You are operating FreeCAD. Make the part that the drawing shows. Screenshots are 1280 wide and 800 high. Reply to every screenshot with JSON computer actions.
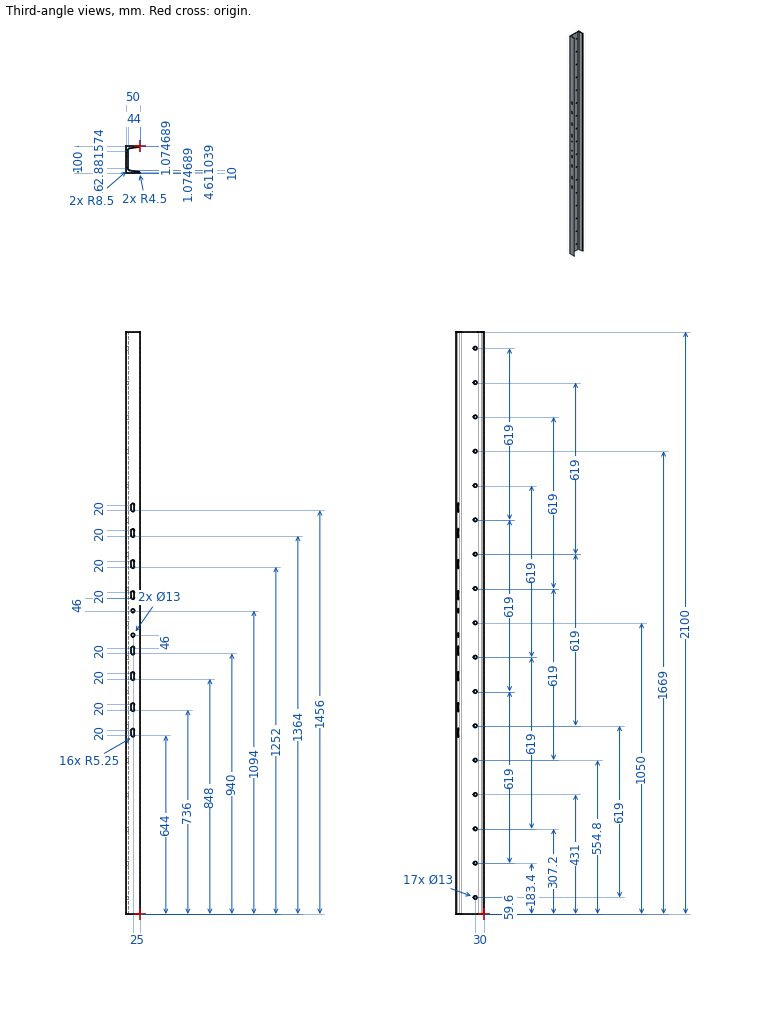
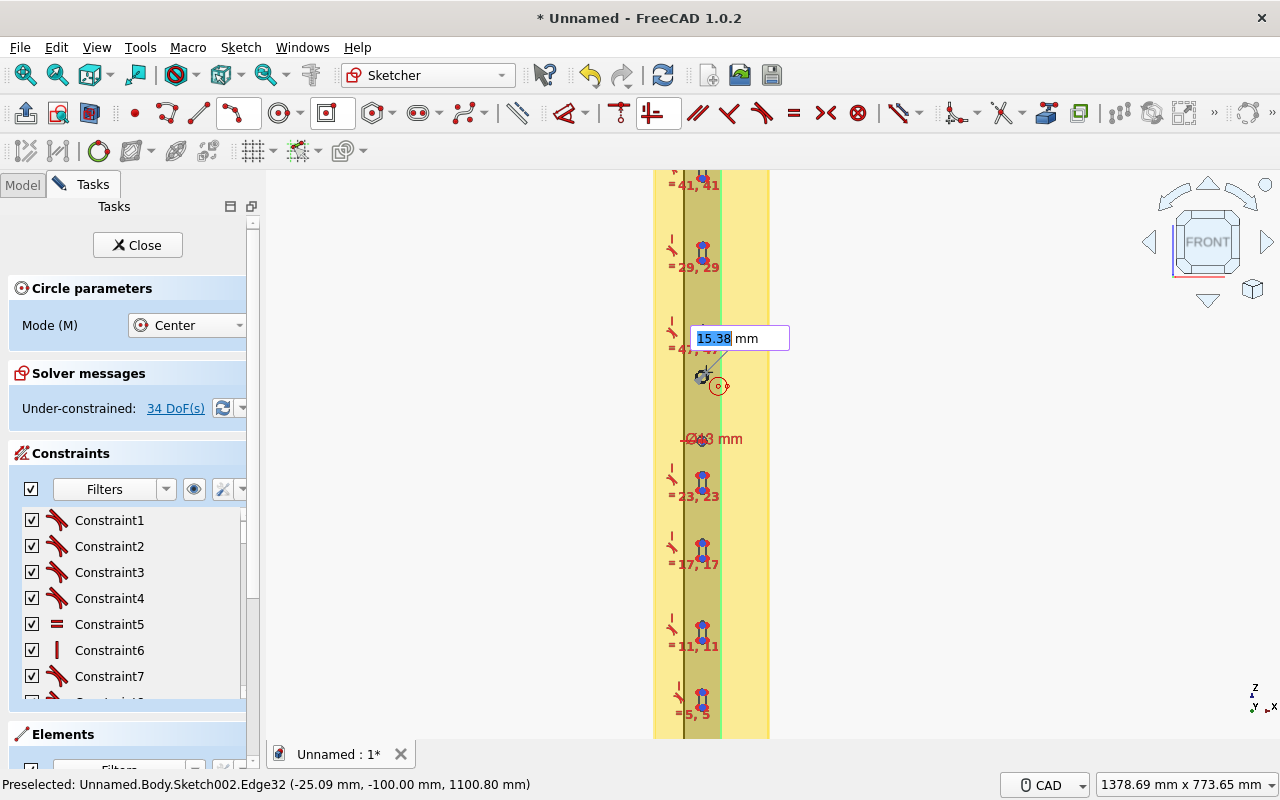
{"action": "type", "text": "13"}
{"action": "key", "text": "Return"}
{"action": "key", "text": "Escape"}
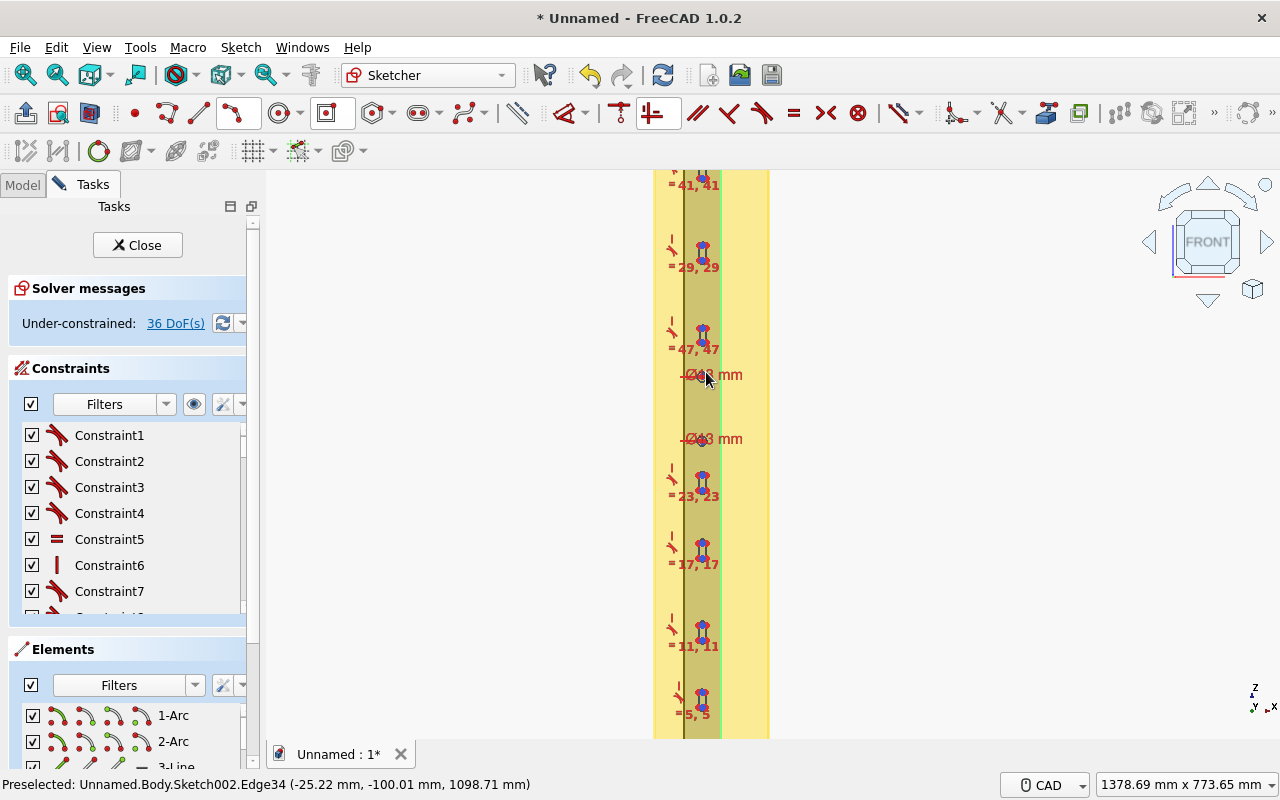
{"action": "scroll", "coordinate": [702, 376], "scroll_direction": "down", "scroll_amount": 6}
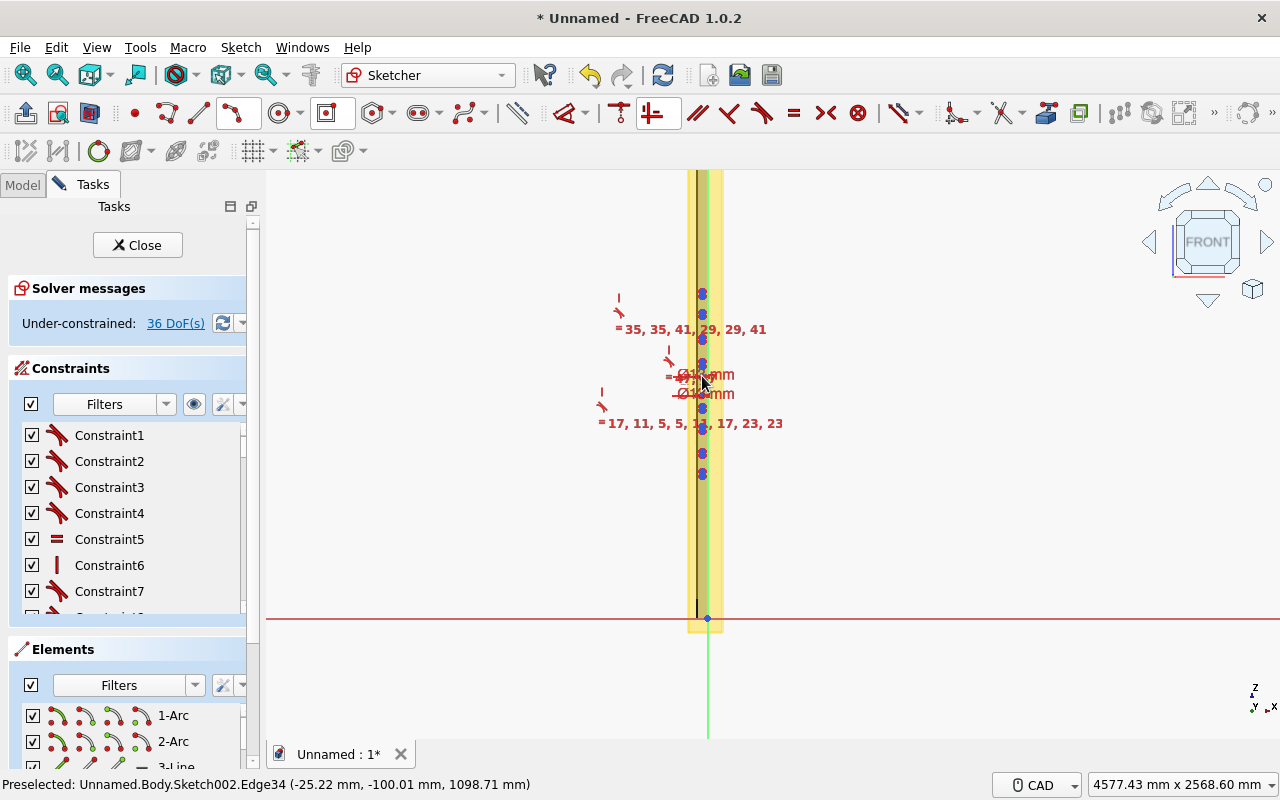
{"action": "scroll", "coordinate": [702, 477], "scroll_direction": "up", "scroll_amount": 13}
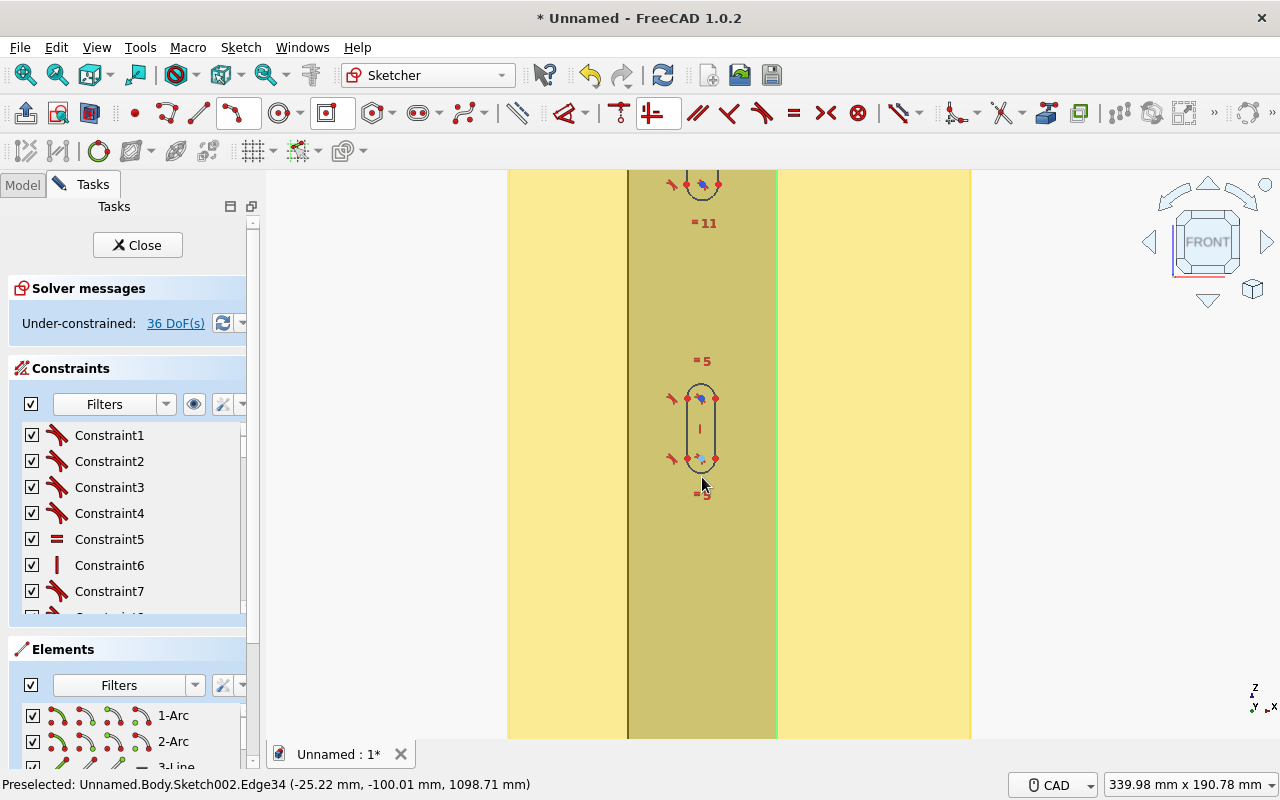
{"action": "left_click", "coordinate": [701, 473]}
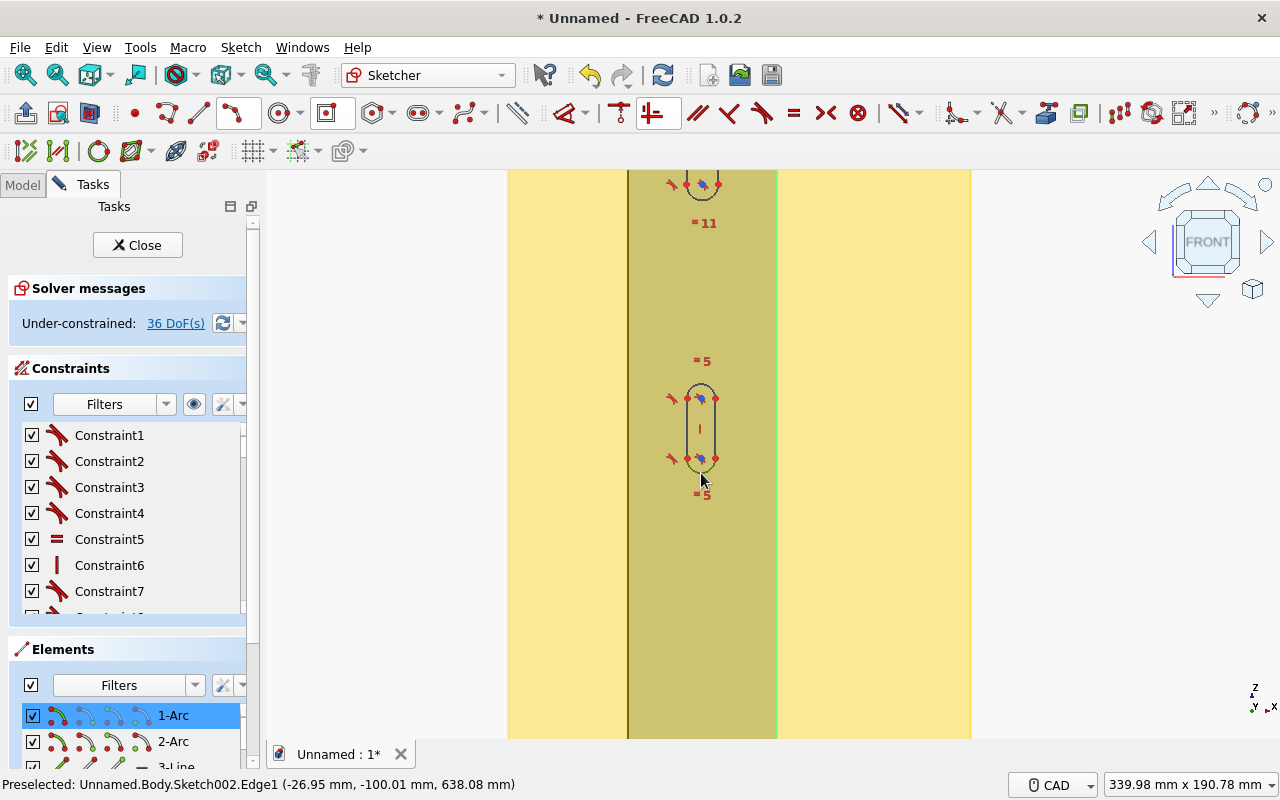
{"action": "left_click", "coordinate": [702, 200]}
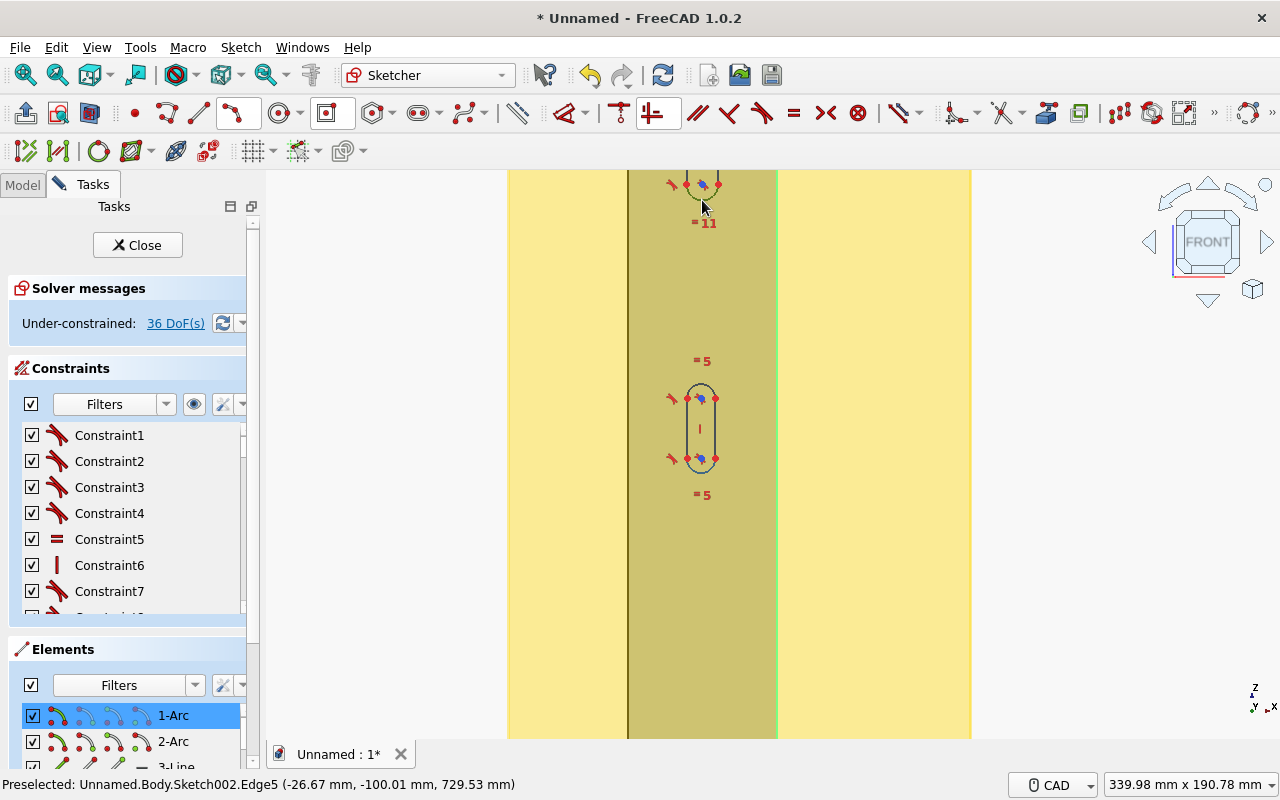
{"action": "scroll", "coordinate": [702, 478], "scroll_direction": "down", "scroll_amount": 13}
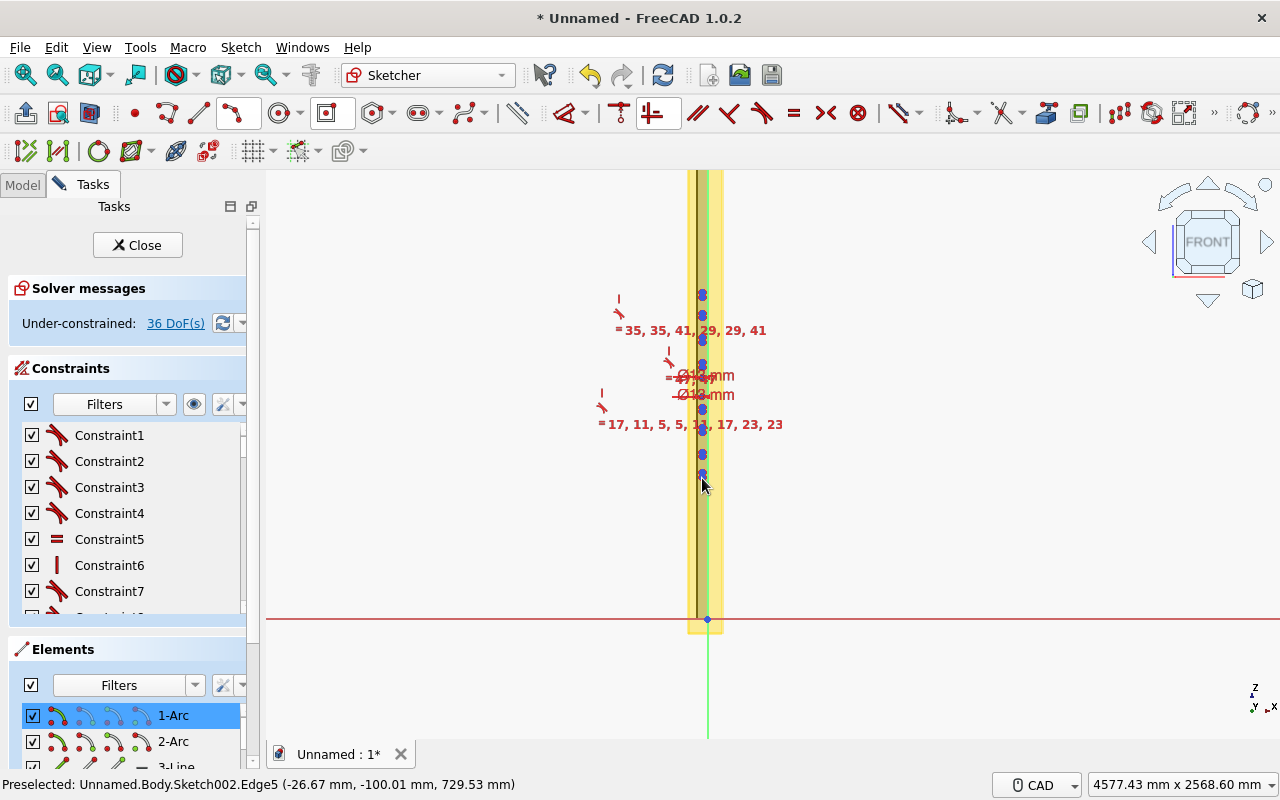
{"action": "scroll", "coordinate": [702, 433], "scroll_direction": "up", "scroll_amount": 14}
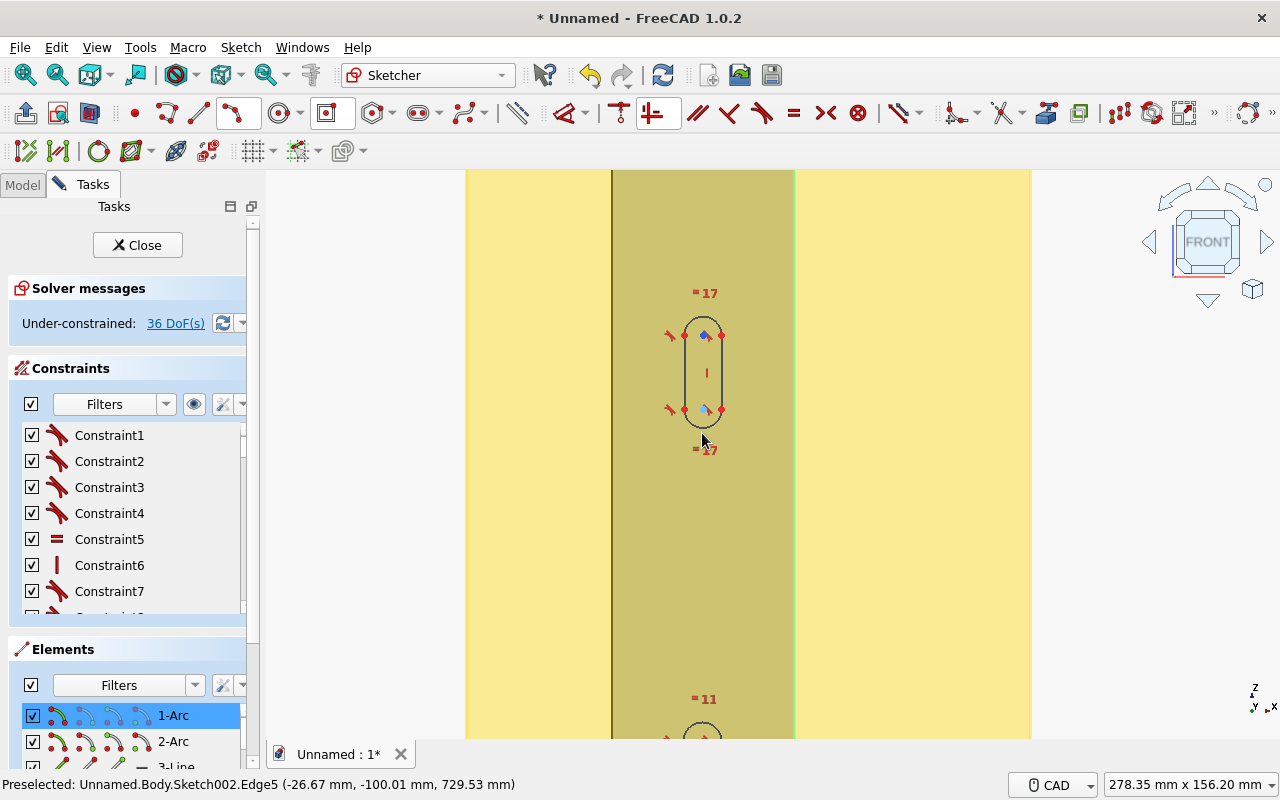
{"action": "left_click", "coordinate": [692, 424]}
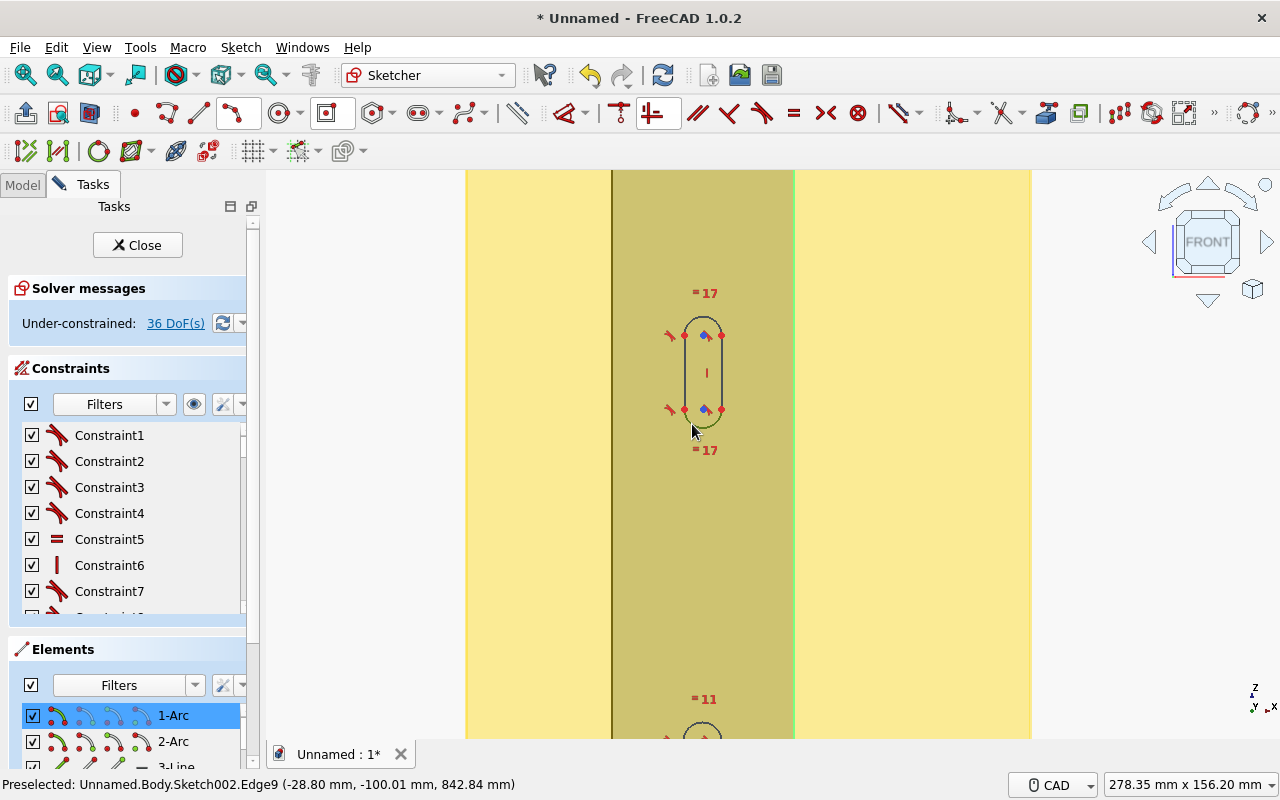
{"action": "scroll", "coordinate": [702, 433], "scroll_direction": "down", "scroll_amount": 14}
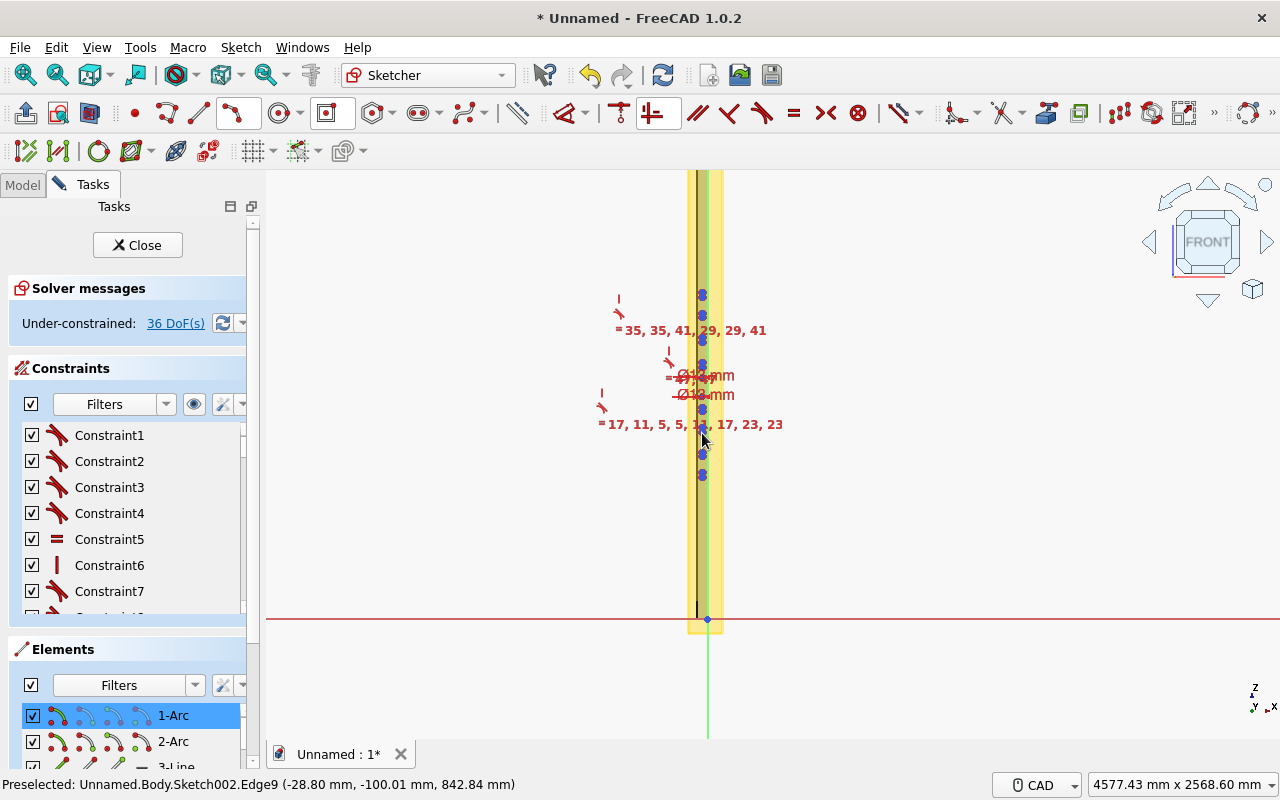
{"action": "scroll", "coordinate": [702, 413], "scroll_direction": "up", "scroll_amount": 14}